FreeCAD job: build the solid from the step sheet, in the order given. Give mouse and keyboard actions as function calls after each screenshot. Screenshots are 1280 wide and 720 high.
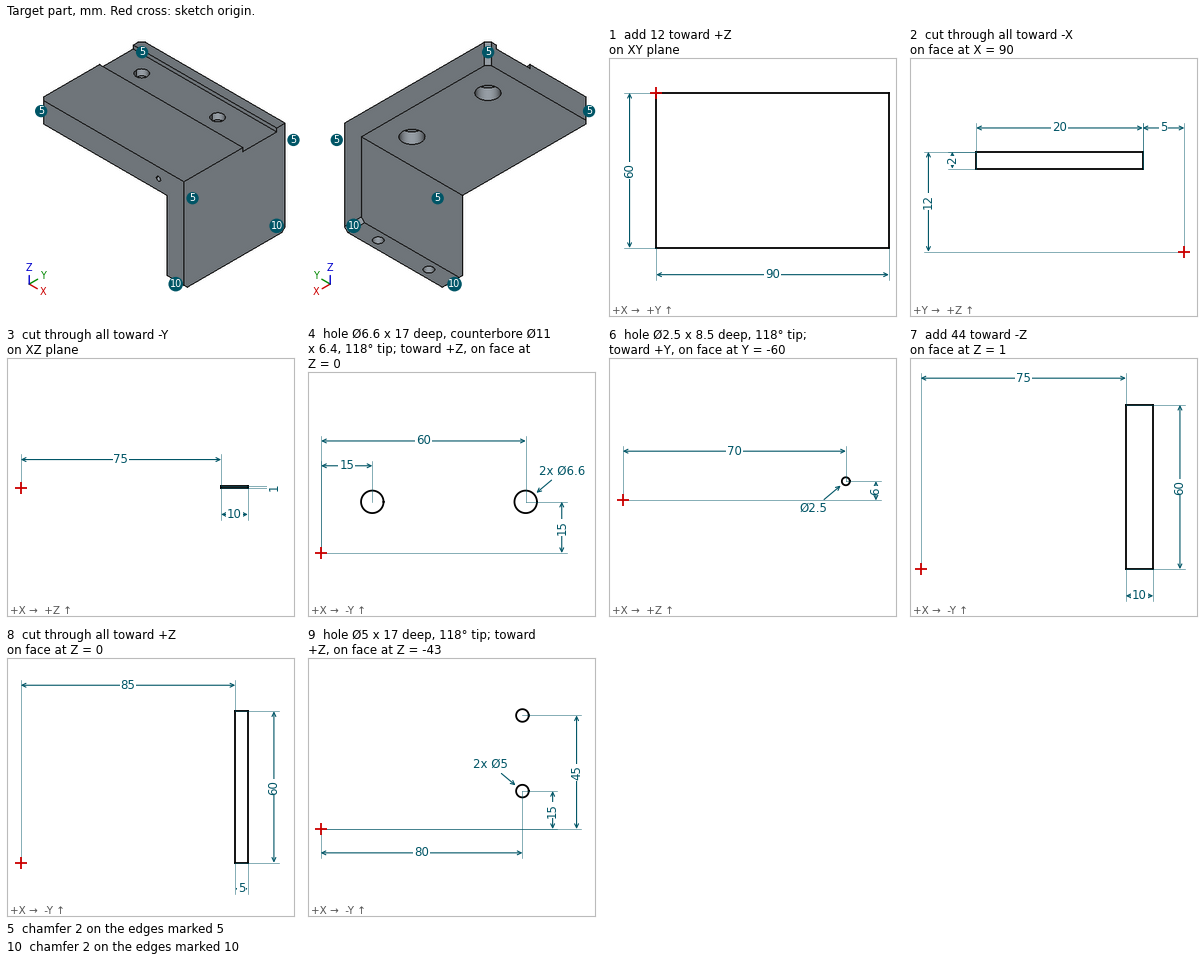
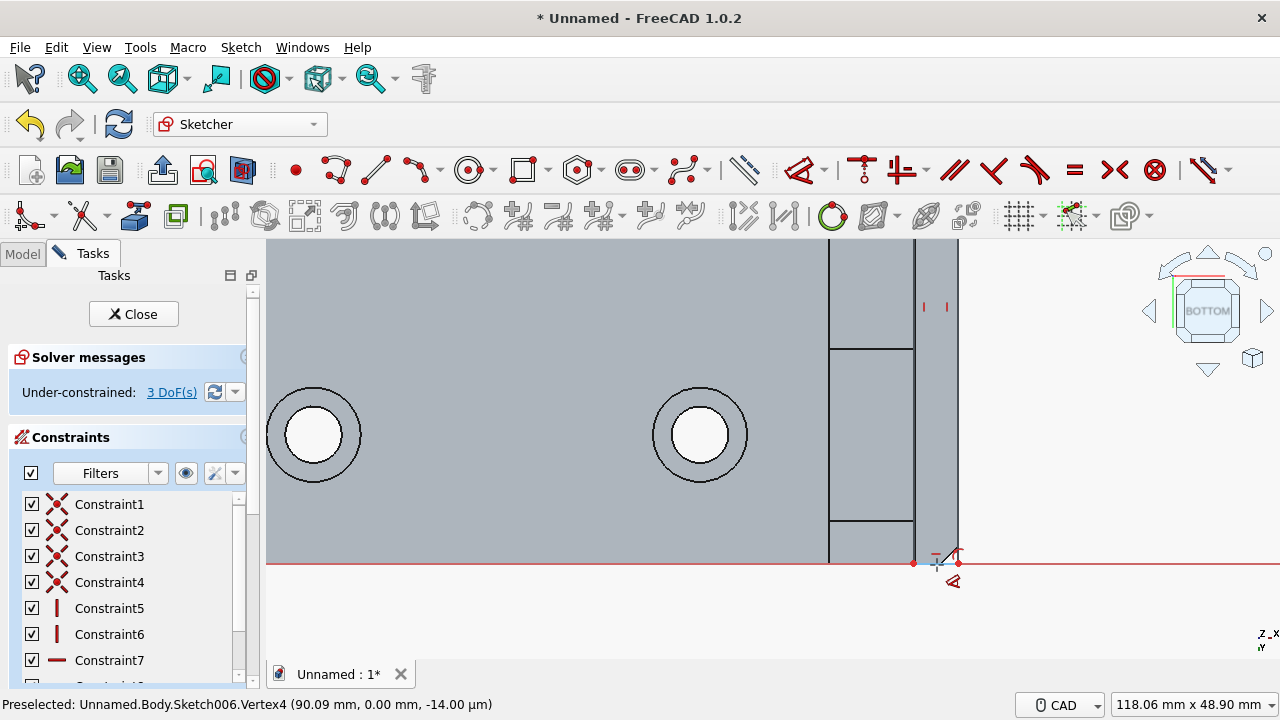
click(936, 564)
click(936, 598)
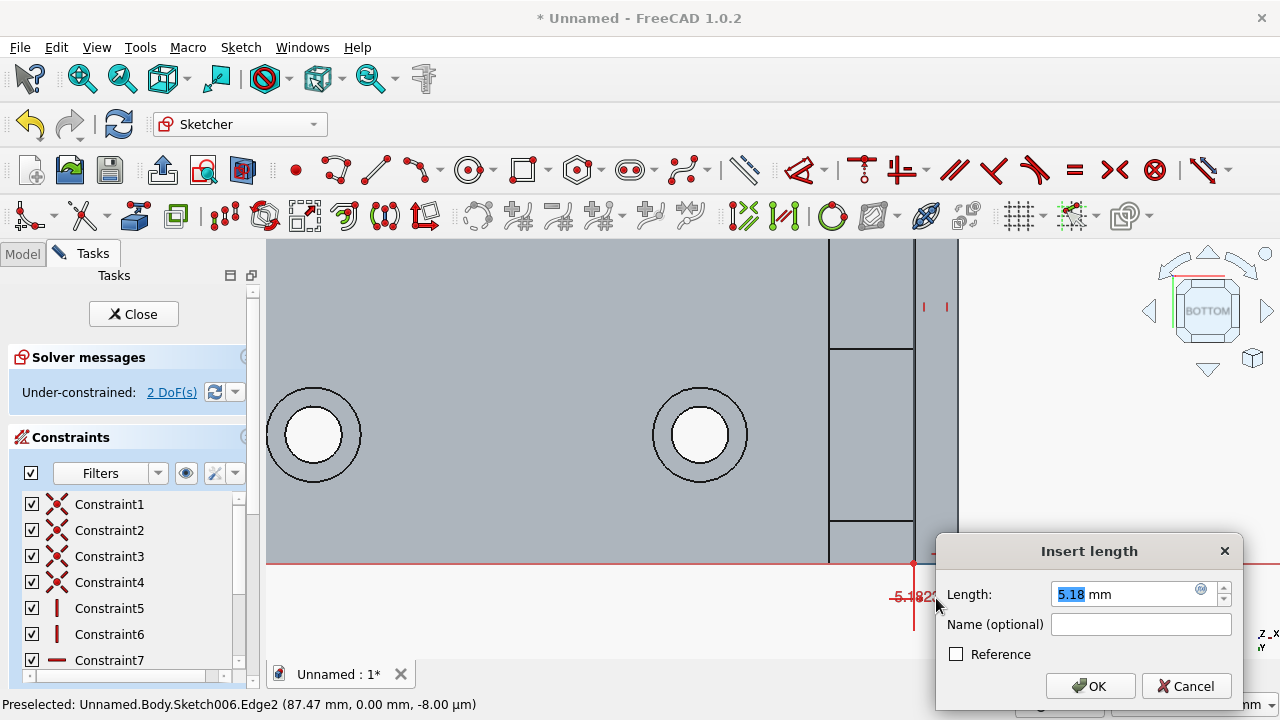
text(5)
key(Return)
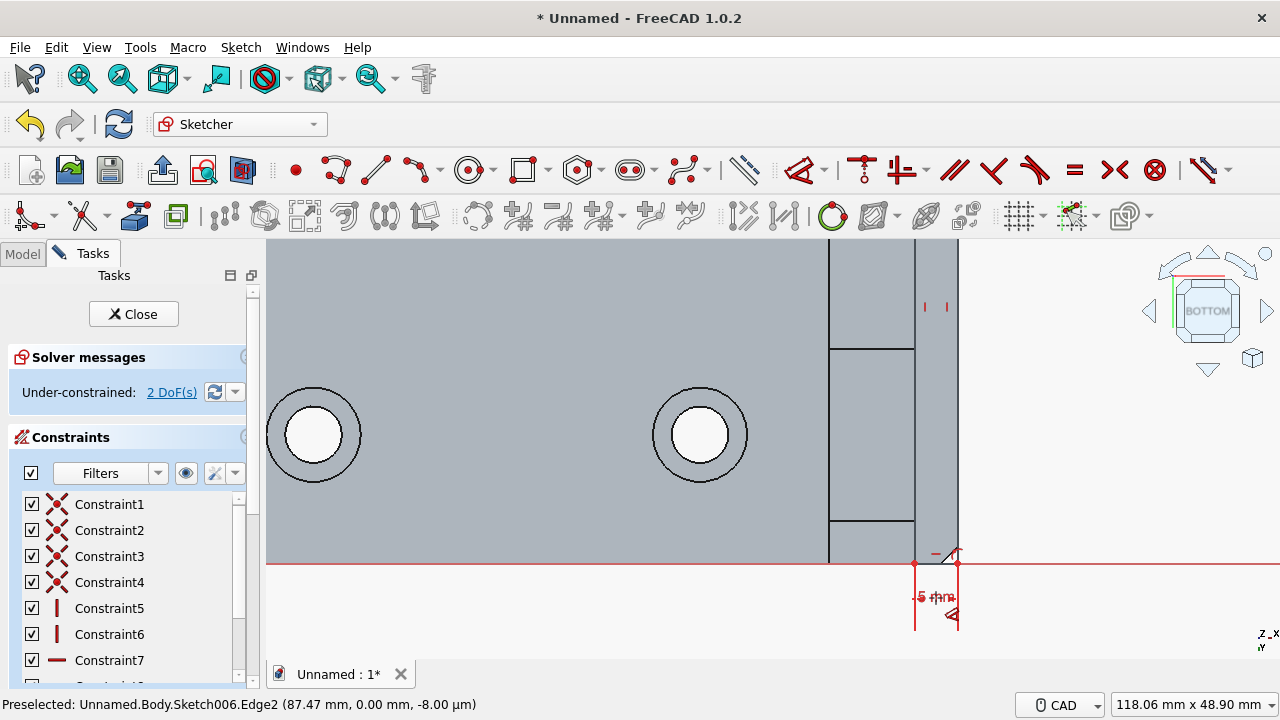
click(915, 409)
click(881, 415)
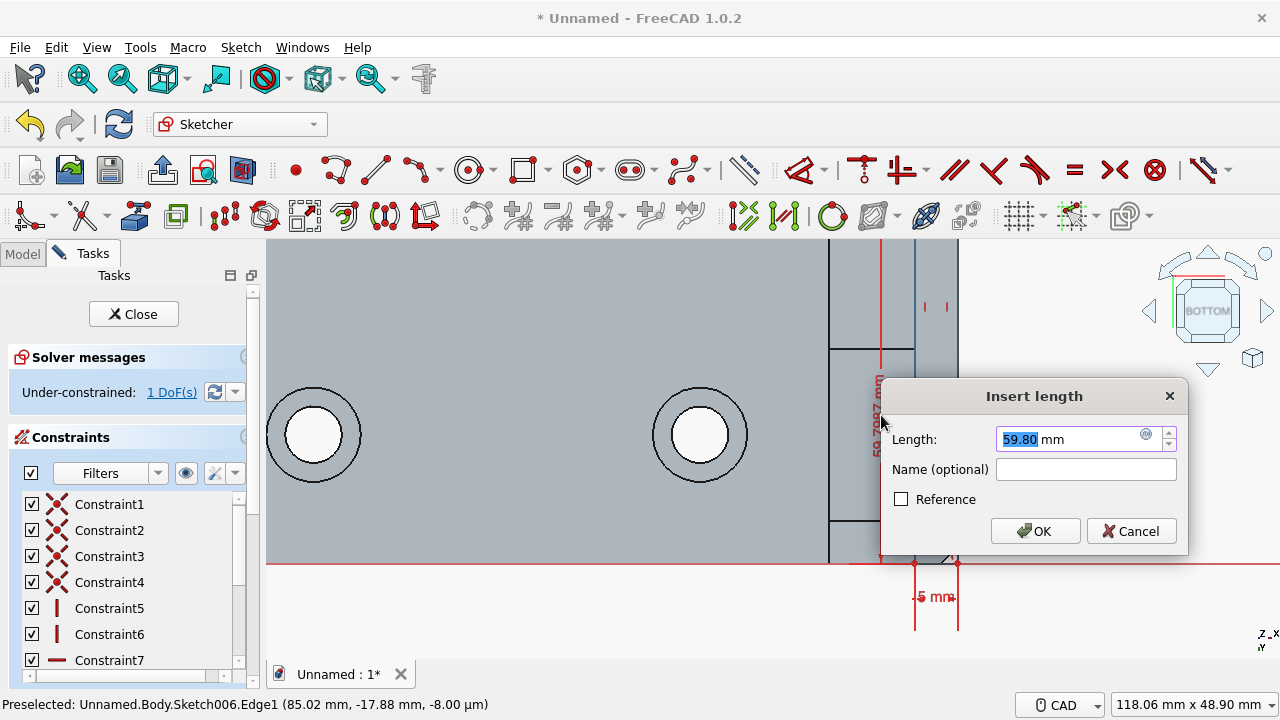
text(60)
key(Return)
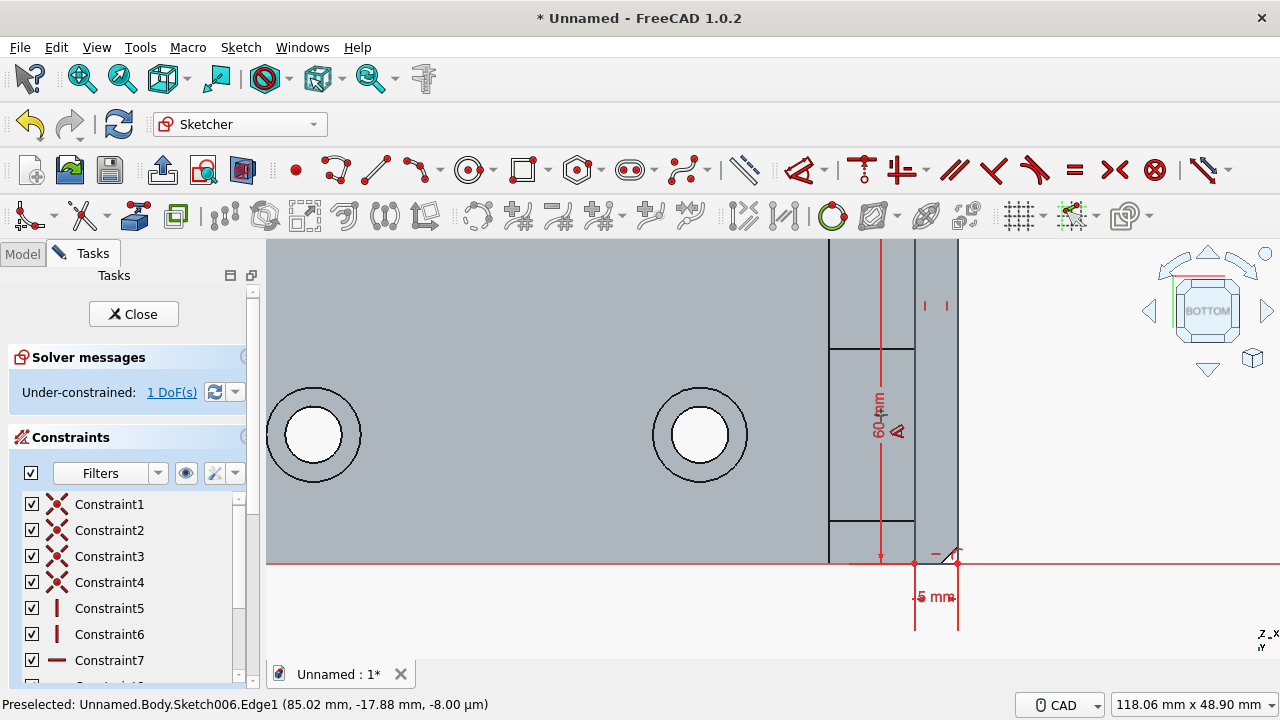
scroll(867, 623, down, 3)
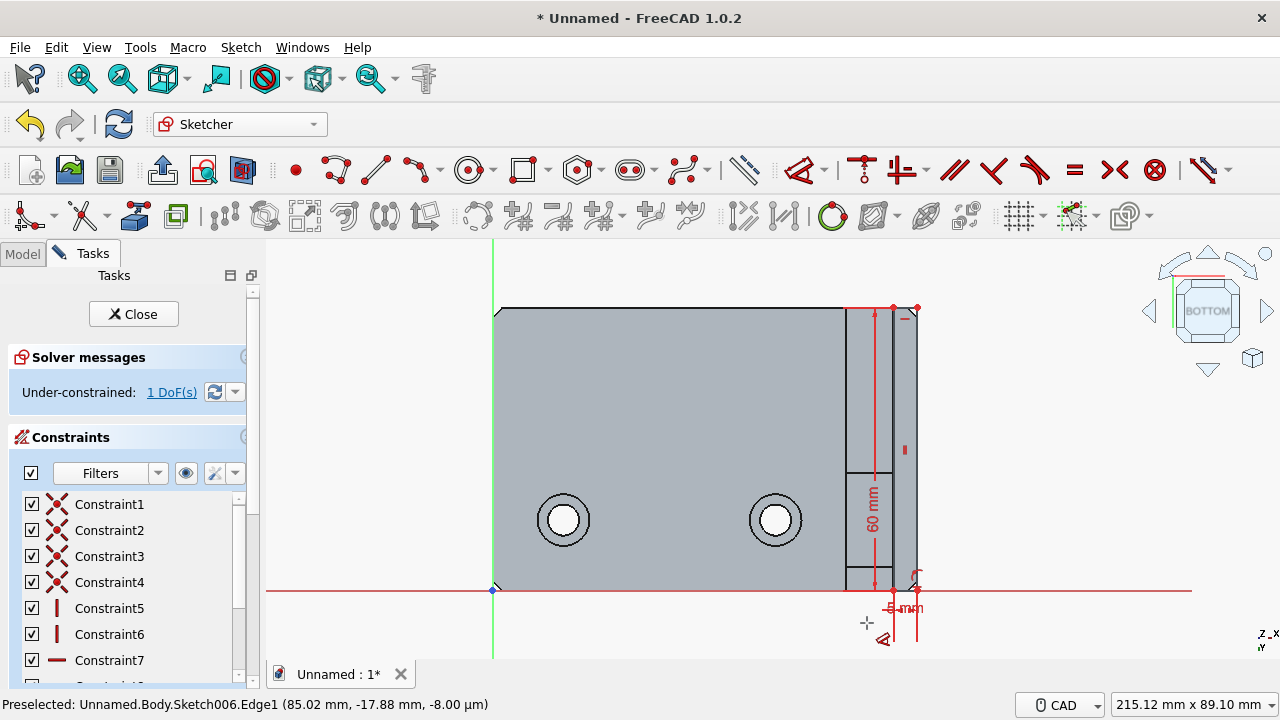
click(894, 308)
click(693, 625)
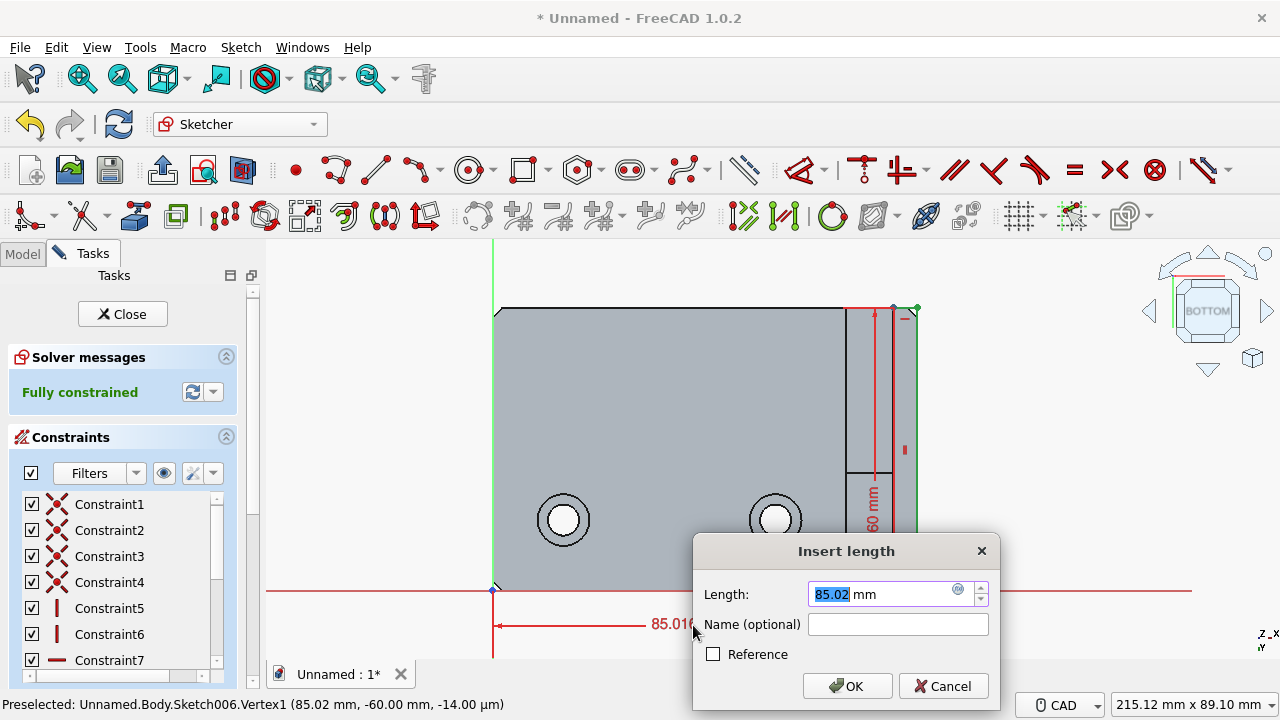
text(85)
key(Return)
key(Escape)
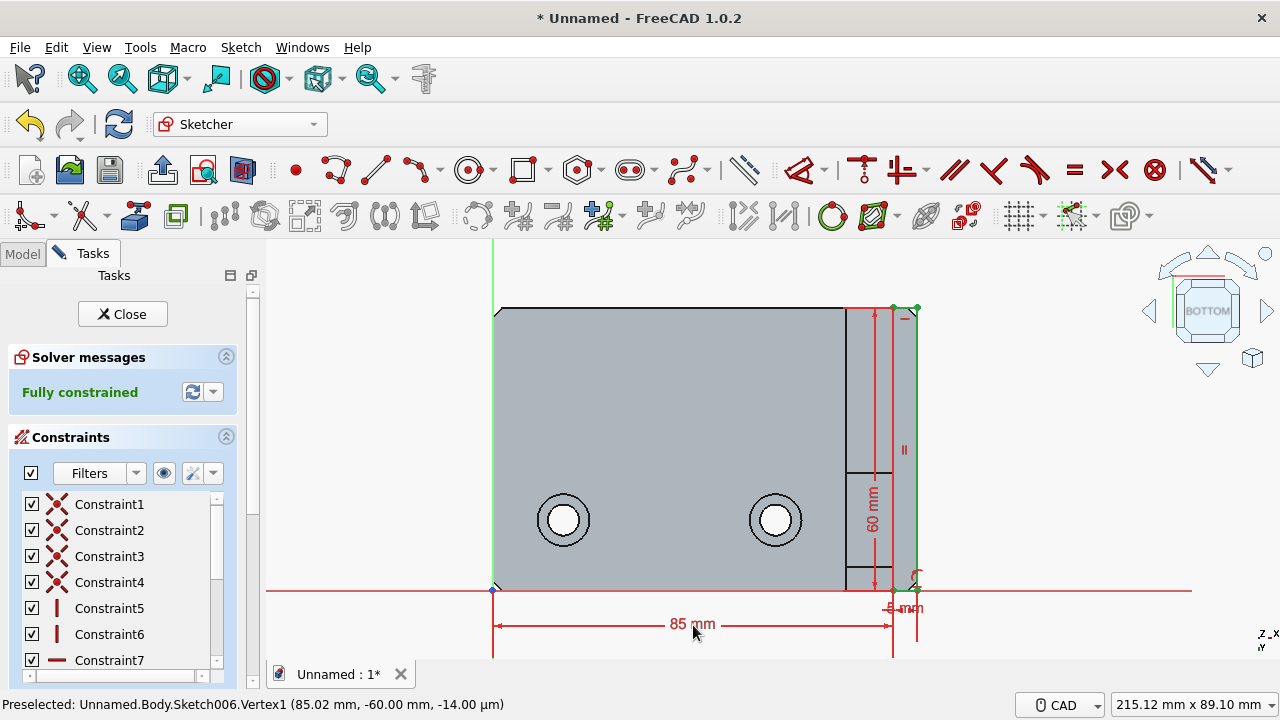
click(123, 314)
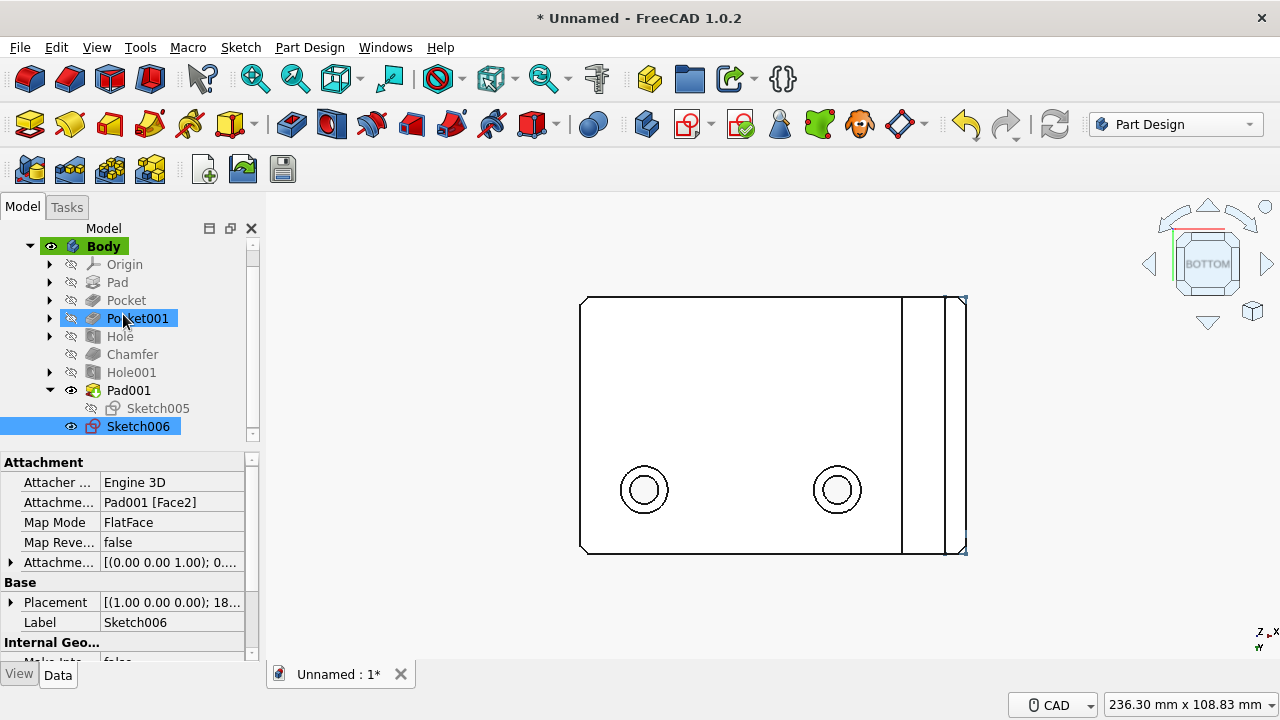
click(292, 124)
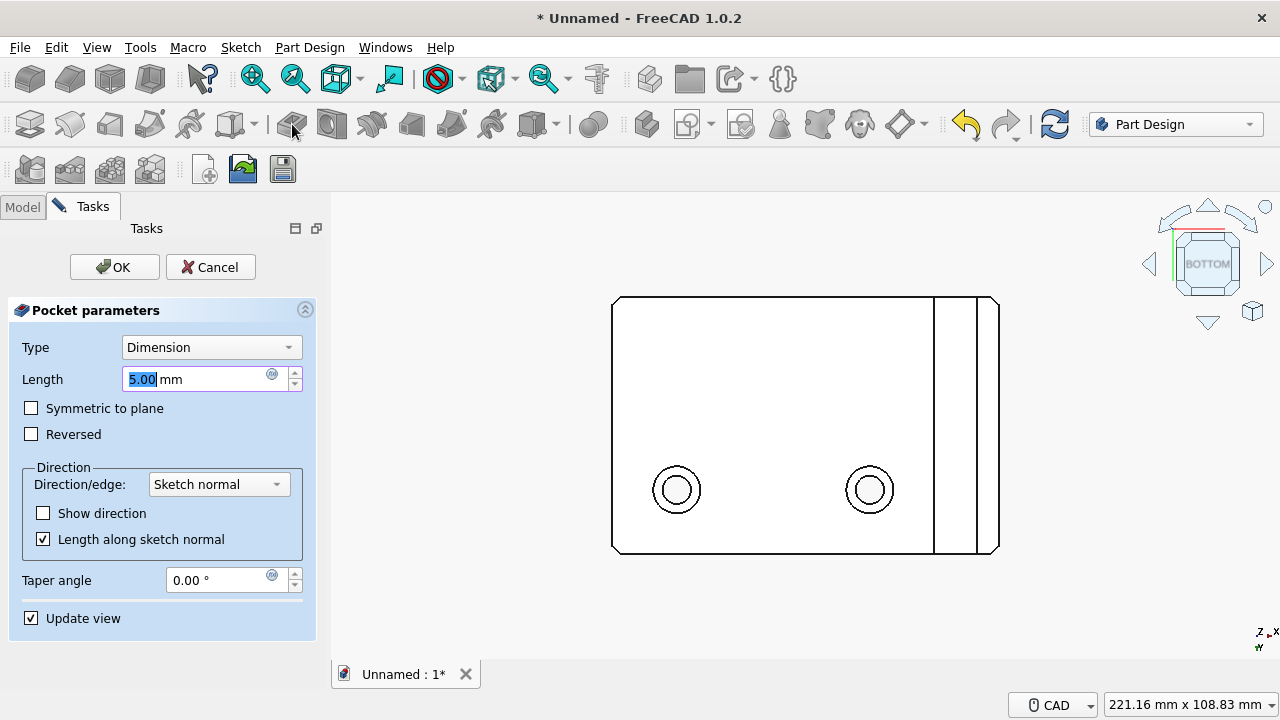
click(212, 348)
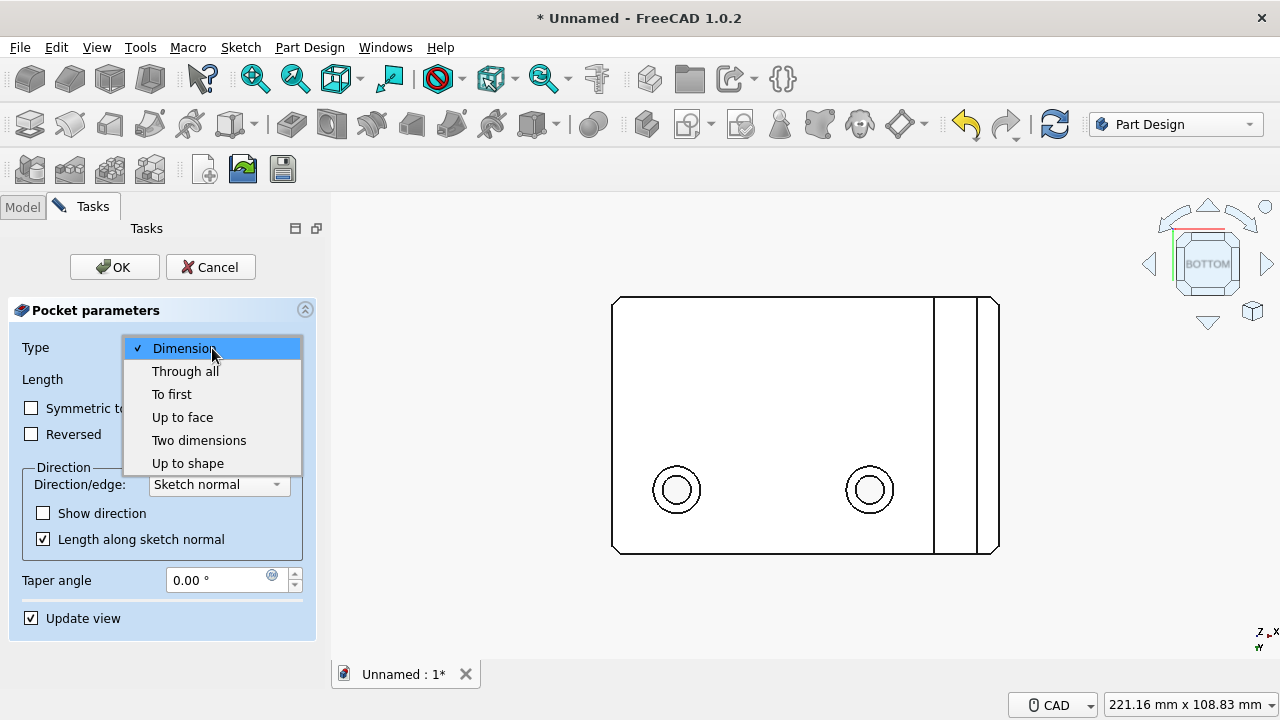
click(212, 372)